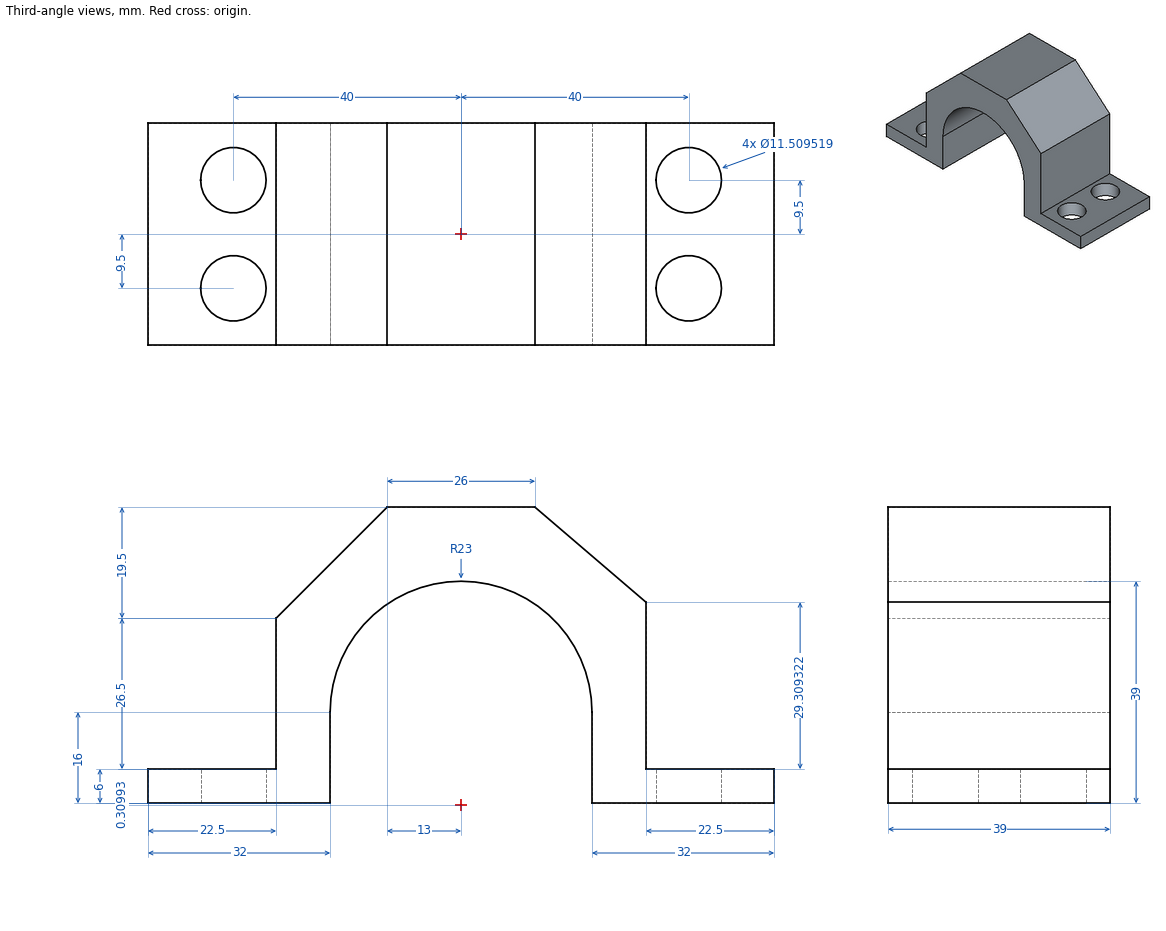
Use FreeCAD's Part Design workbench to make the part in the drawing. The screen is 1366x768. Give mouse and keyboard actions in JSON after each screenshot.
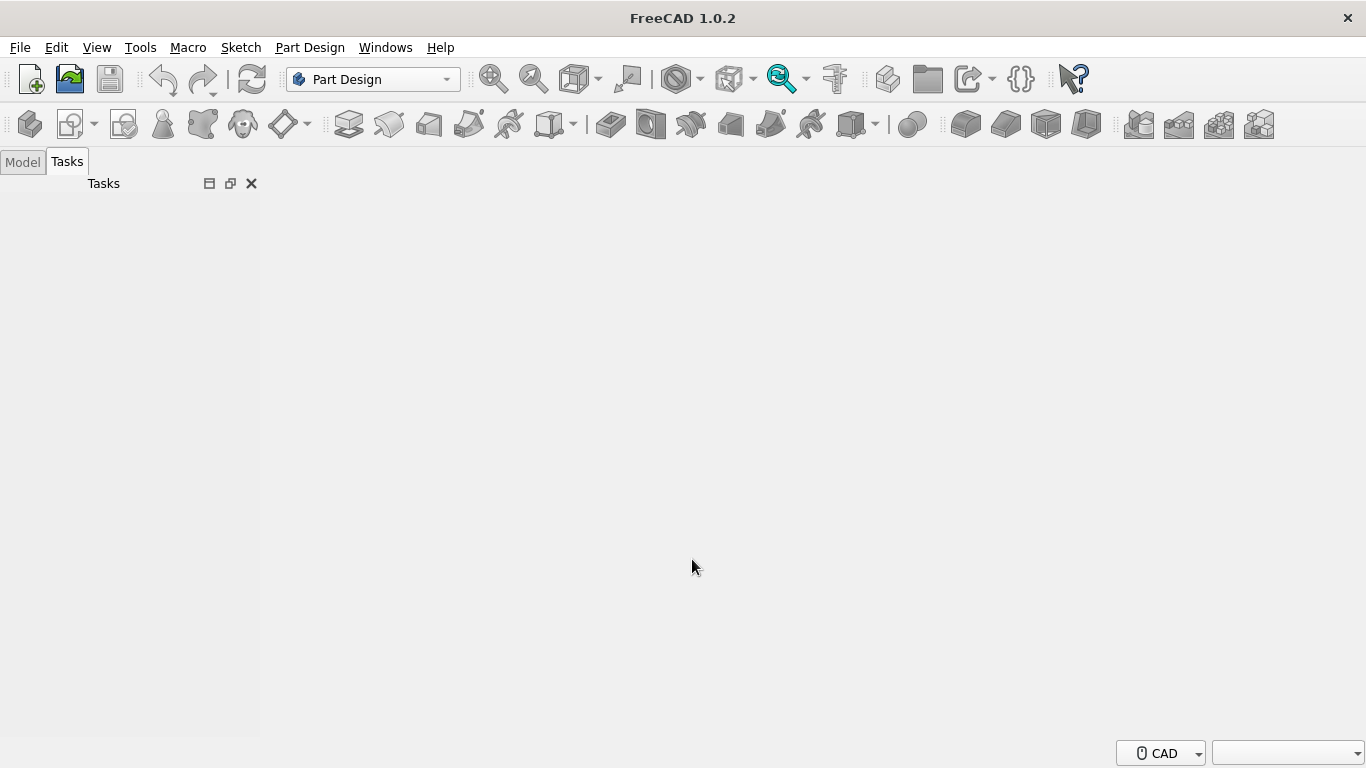
{"action": "key", "text": "ctrl+n"}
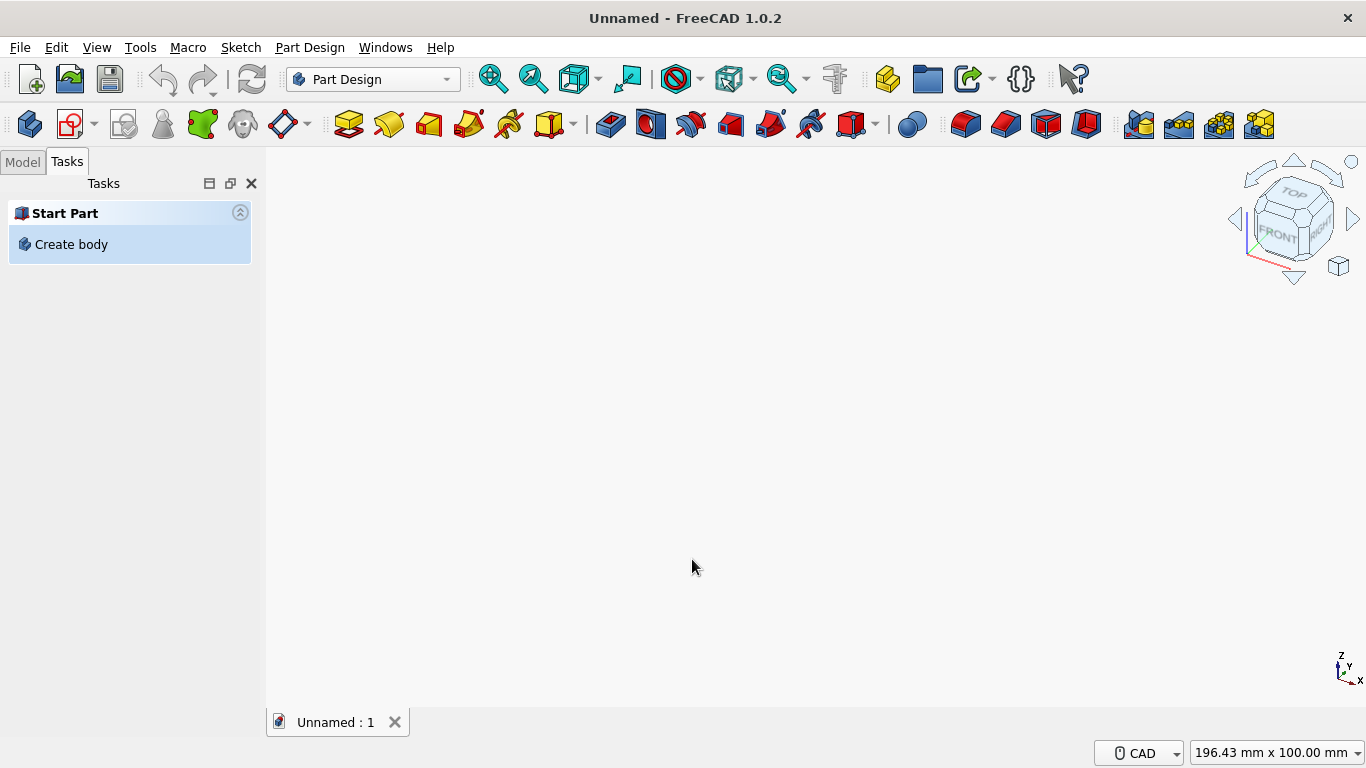
{"action": "left_click", "coordinate": [70, 124]}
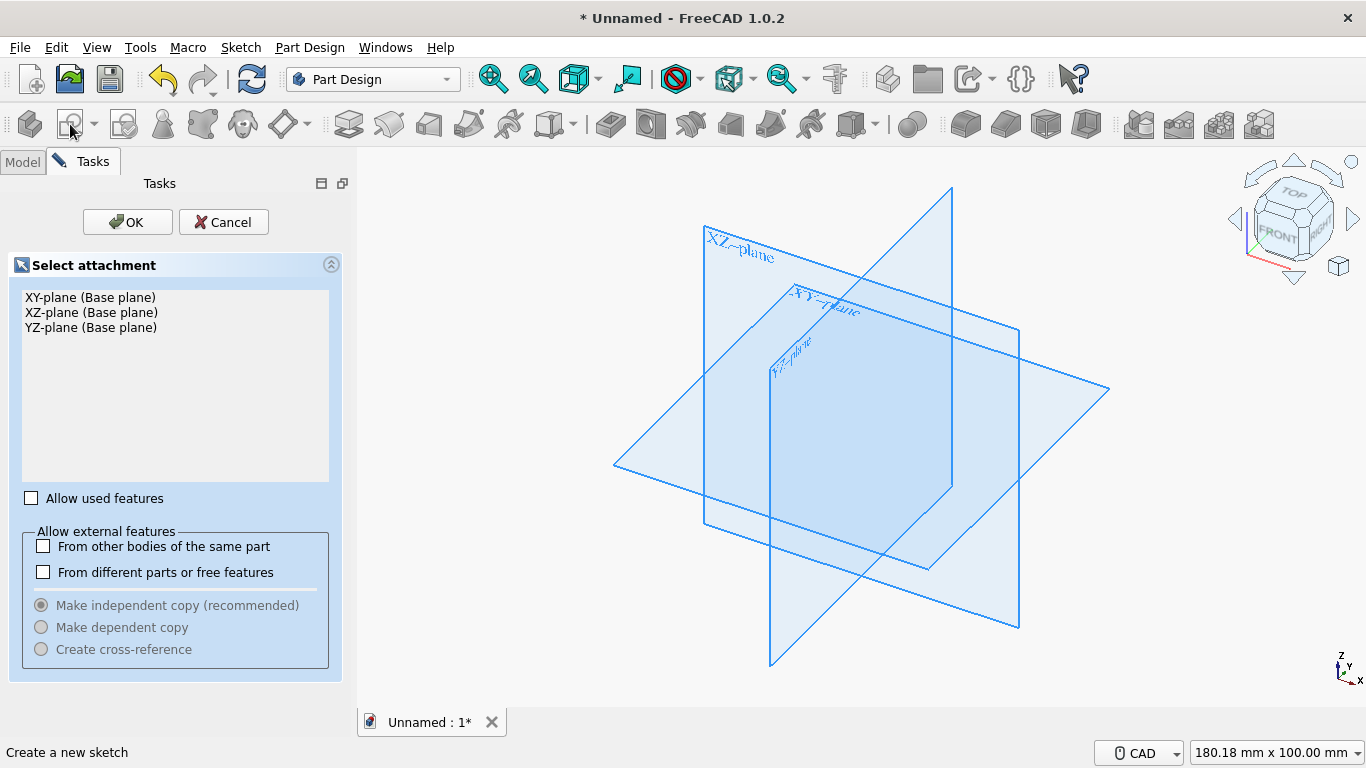
{"action": "left_click", "coordinate": [82, 312]}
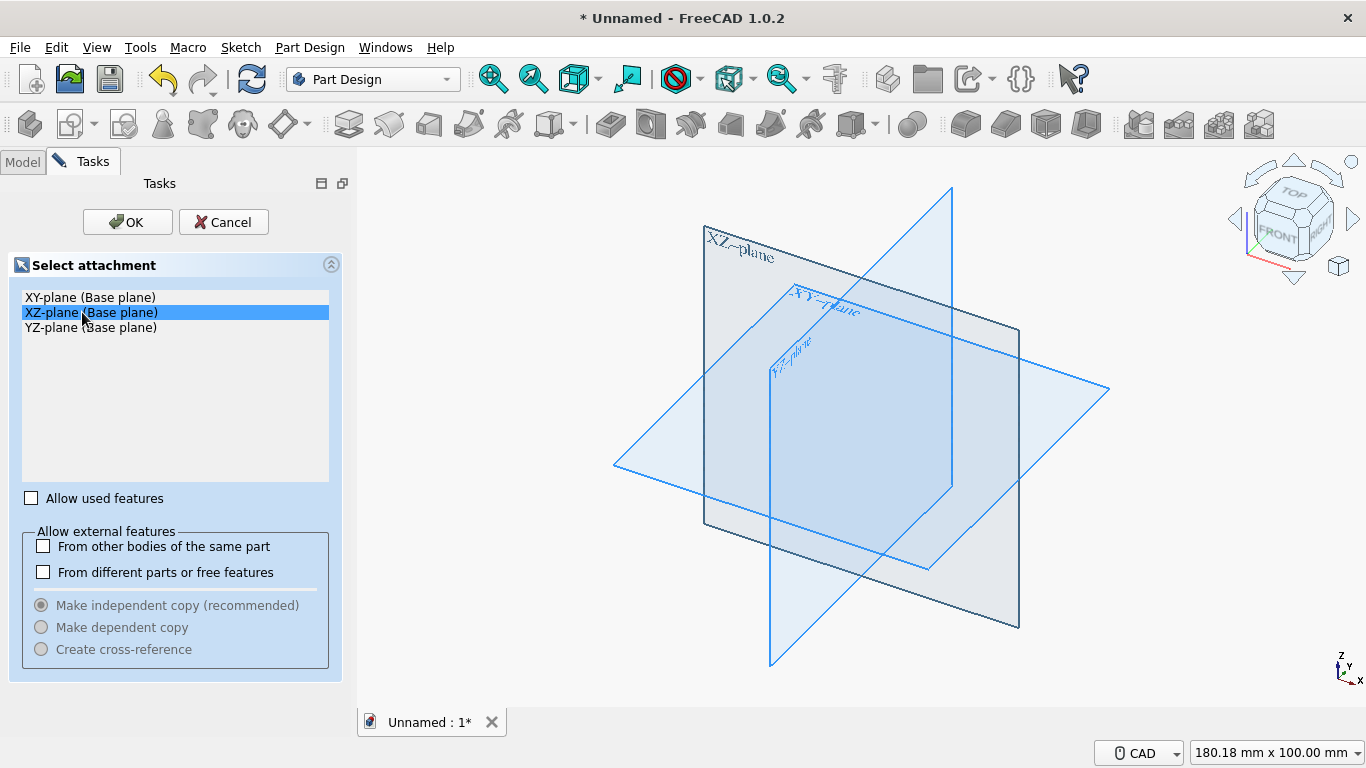
{"action": "left_click", "coordinate": [128, 222]}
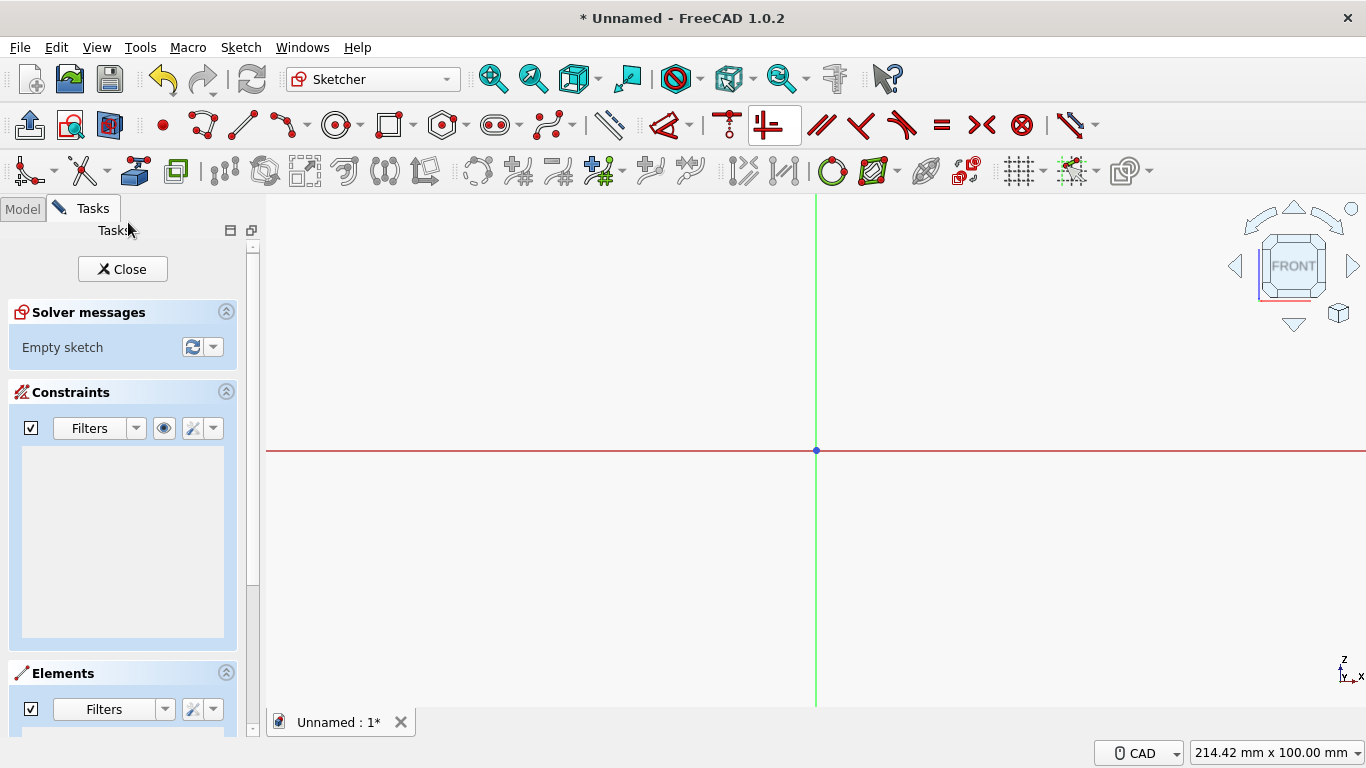
{"action": "scroll", "coordinate": [438, 679], "scroll_direction": "down", "scroll_amount": 1}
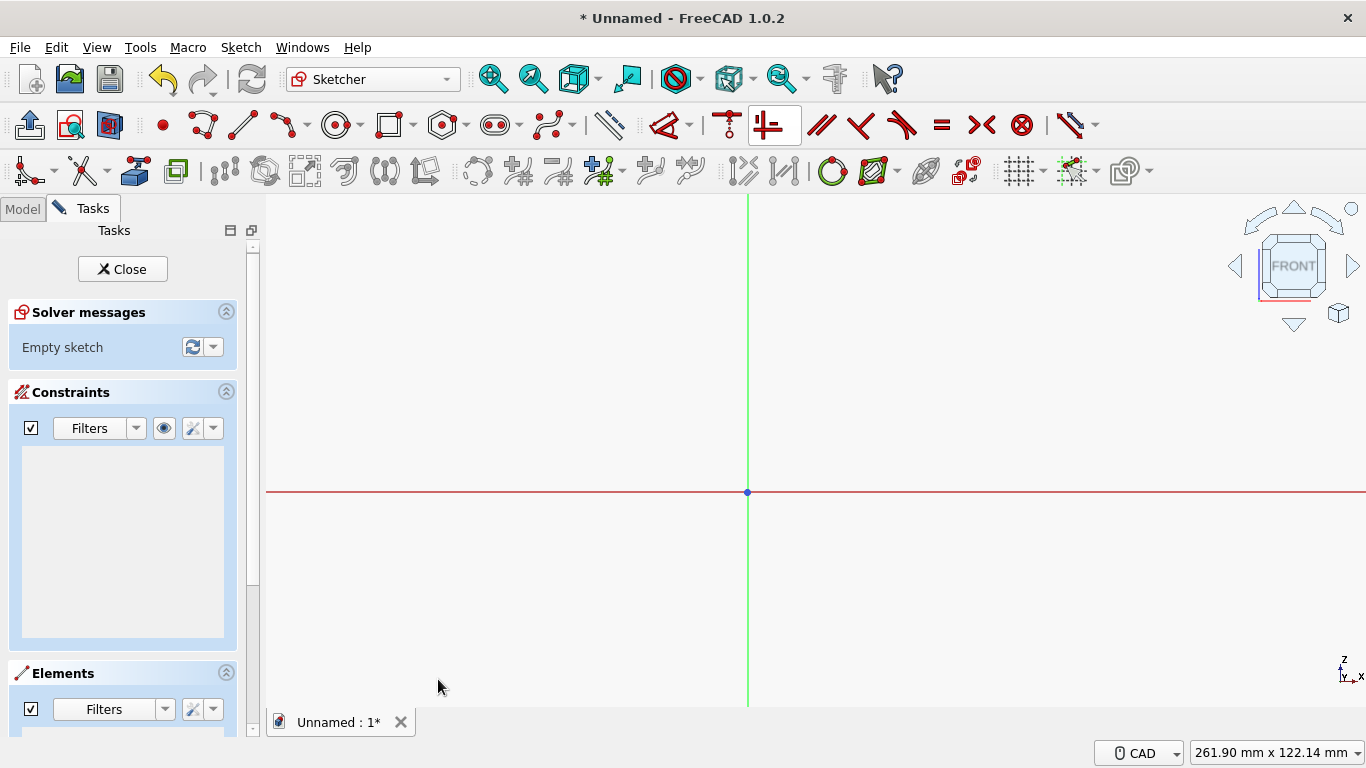
{"action": "scroll", "coordinate": [748, 243], "scroll_direction": "up", "scroll_amount": 2}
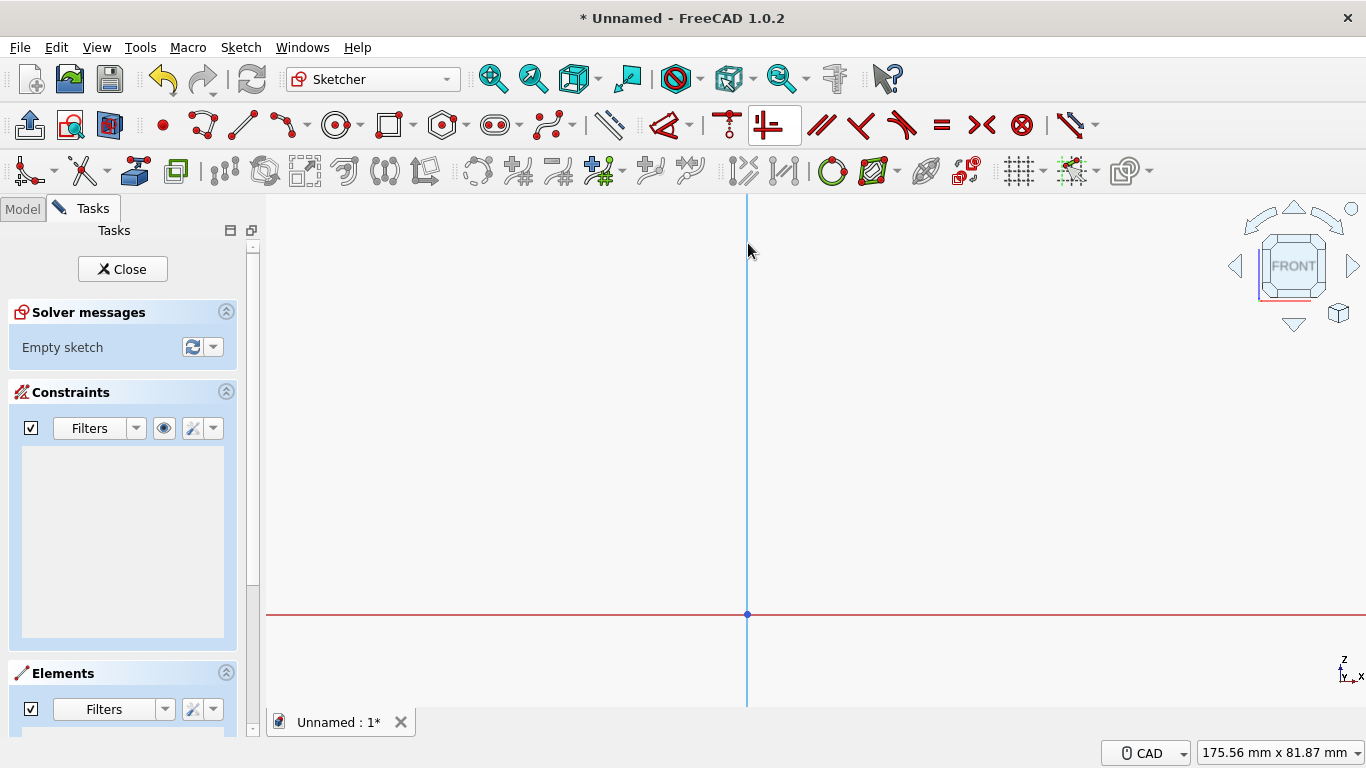
{"action": "key", "text": "g m"}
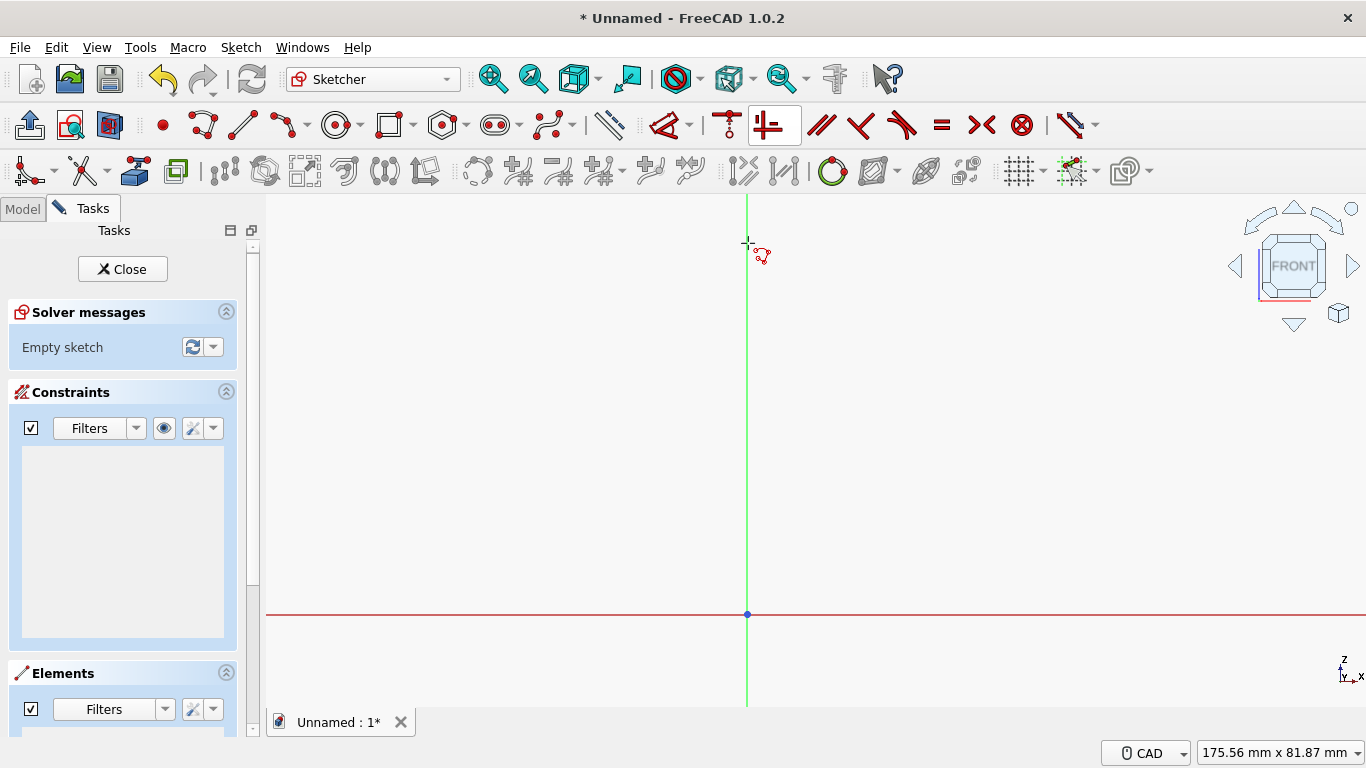
{"action": "left_click", "coordinate": [603, 512]}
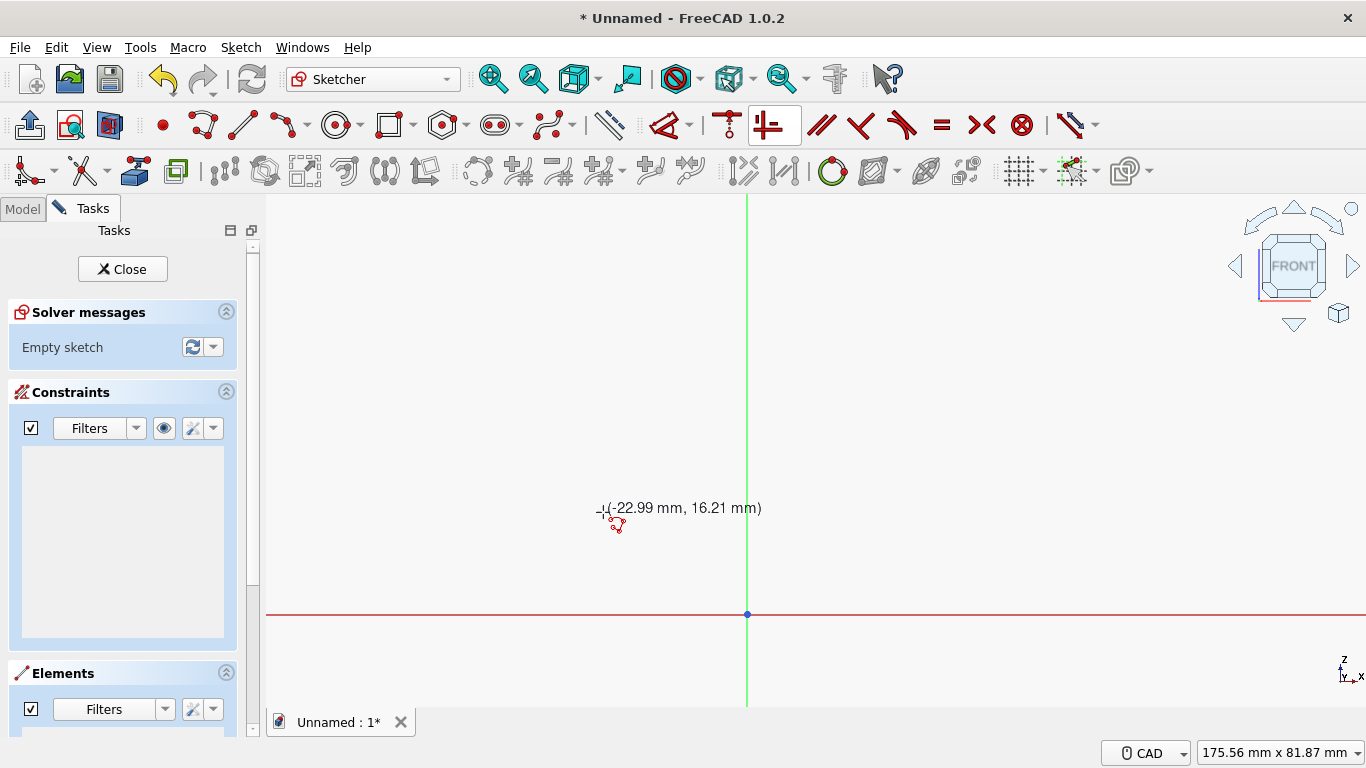
{"action": "scroll", "coordinate": [603, 613], "scroll_direction": "up", "scroll_amount": 11}